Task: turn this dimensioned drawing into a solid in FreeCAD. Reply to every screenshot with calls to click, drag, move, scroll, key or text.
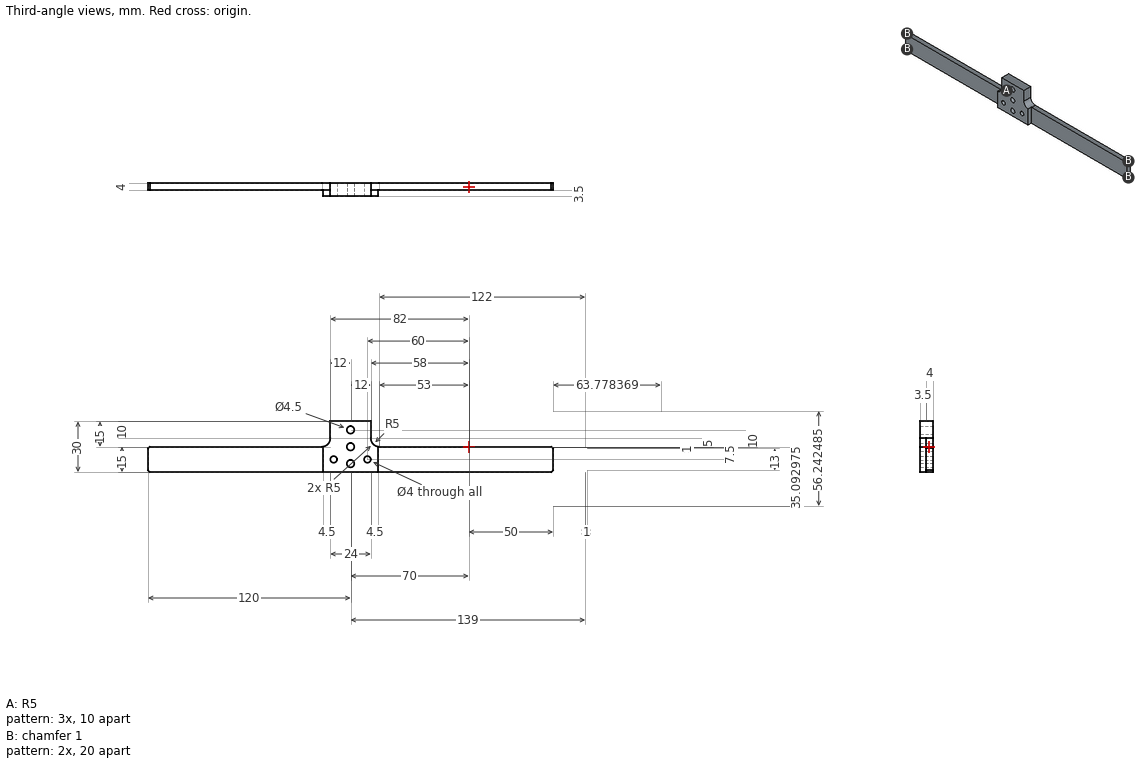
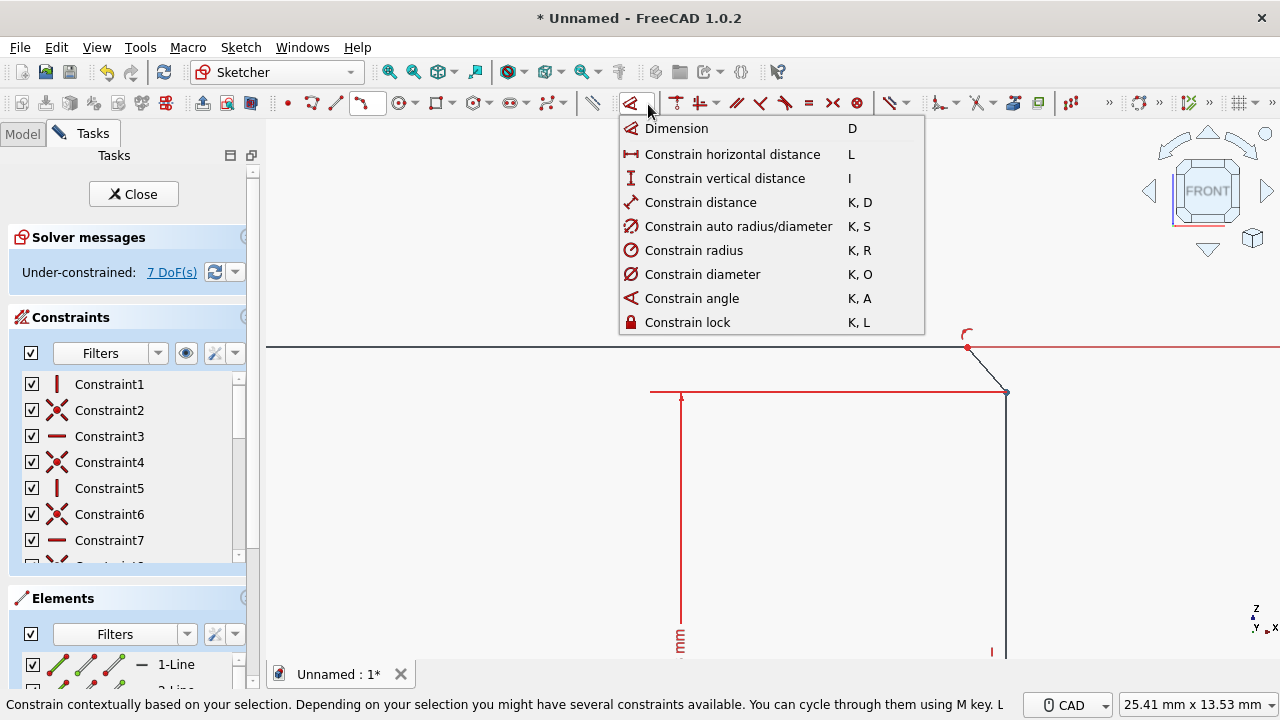
click(772, 178)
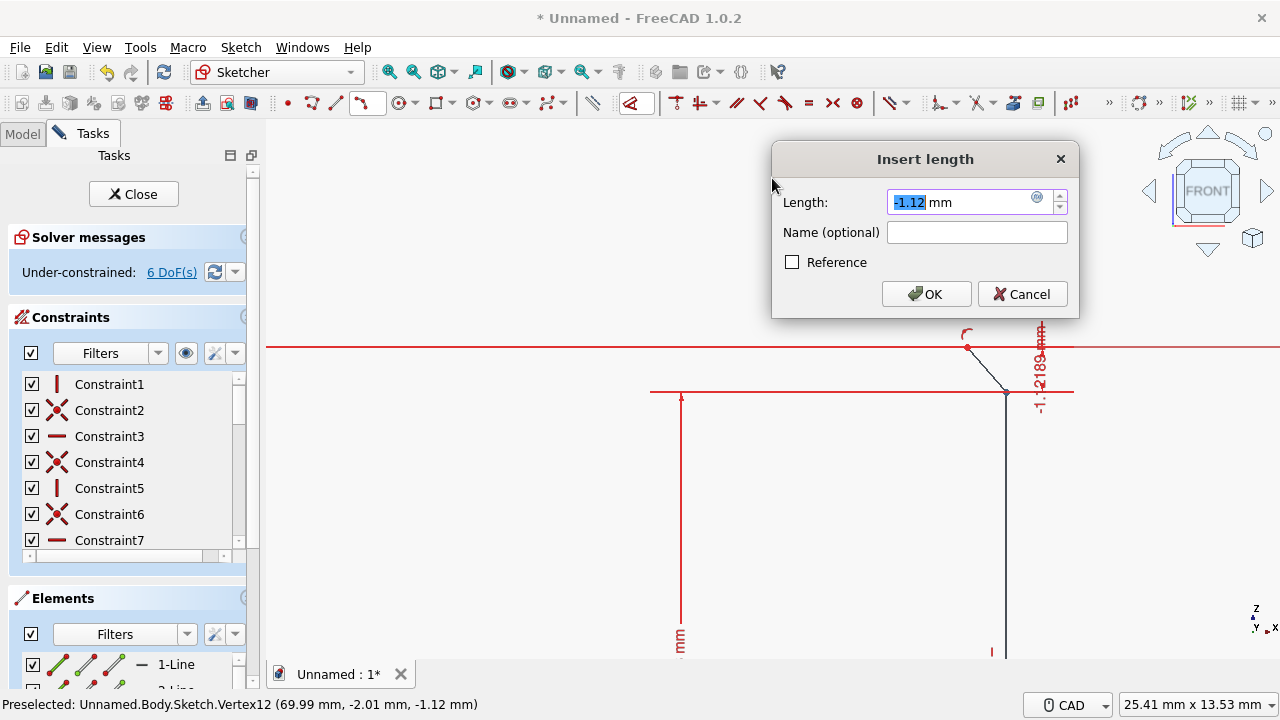
text(-1)
key(Return)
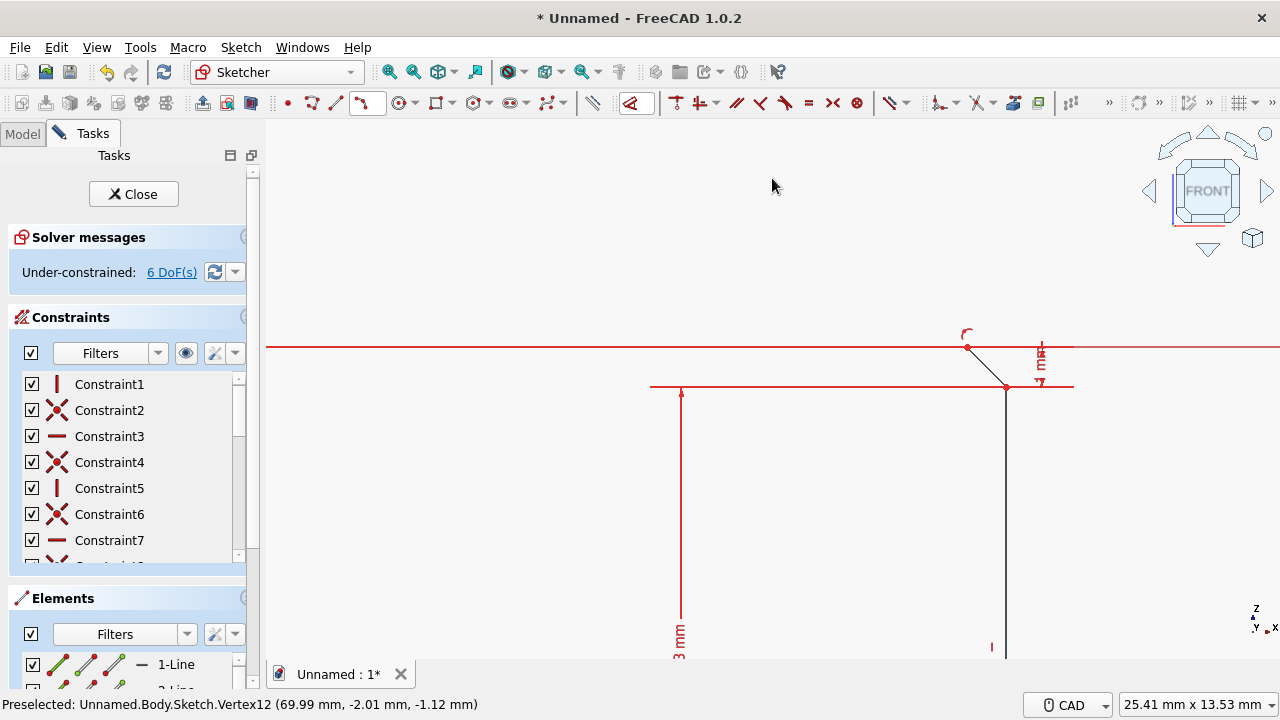
scroll(1015, 394, down, 11)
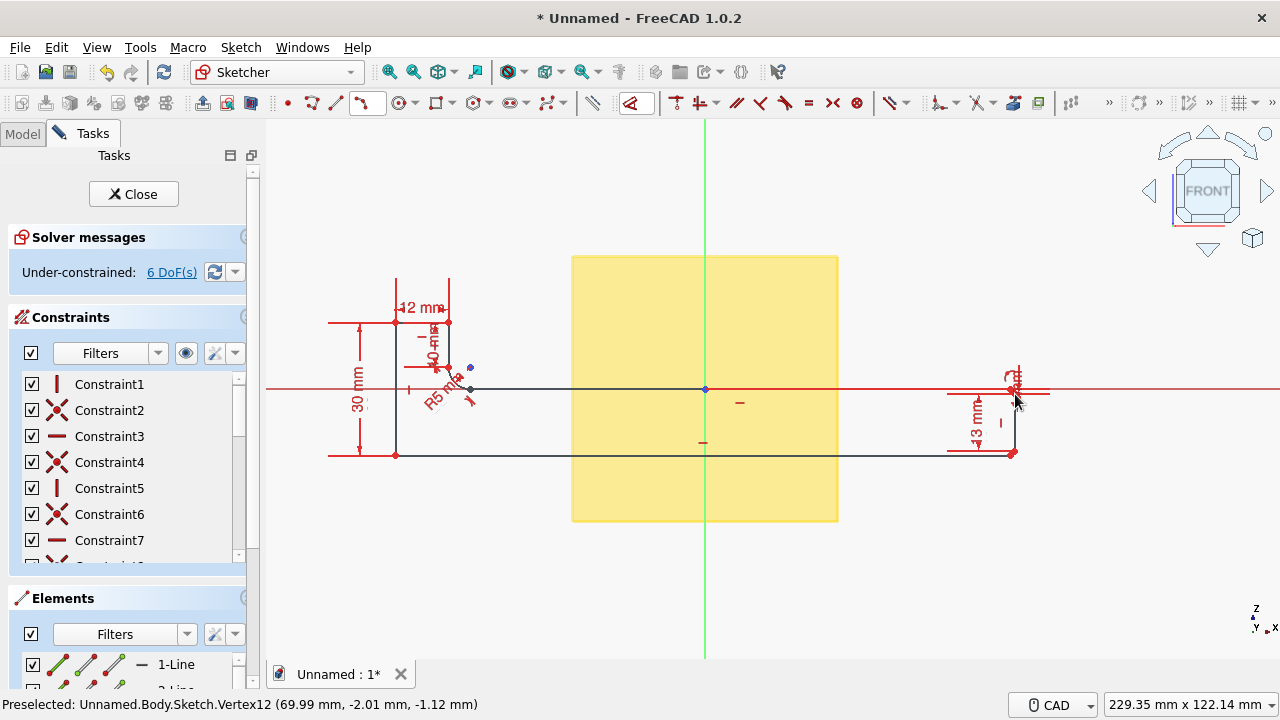
scroll(1012, 454, up, 11)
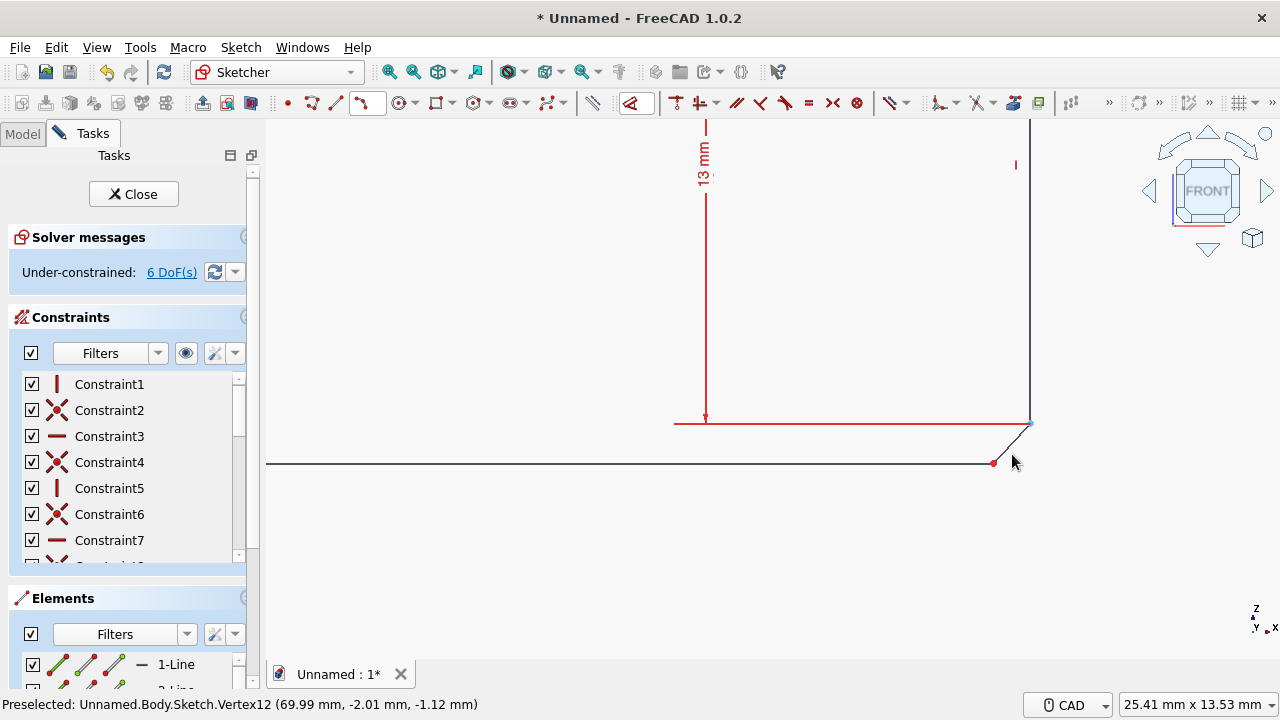
click(1005, 452)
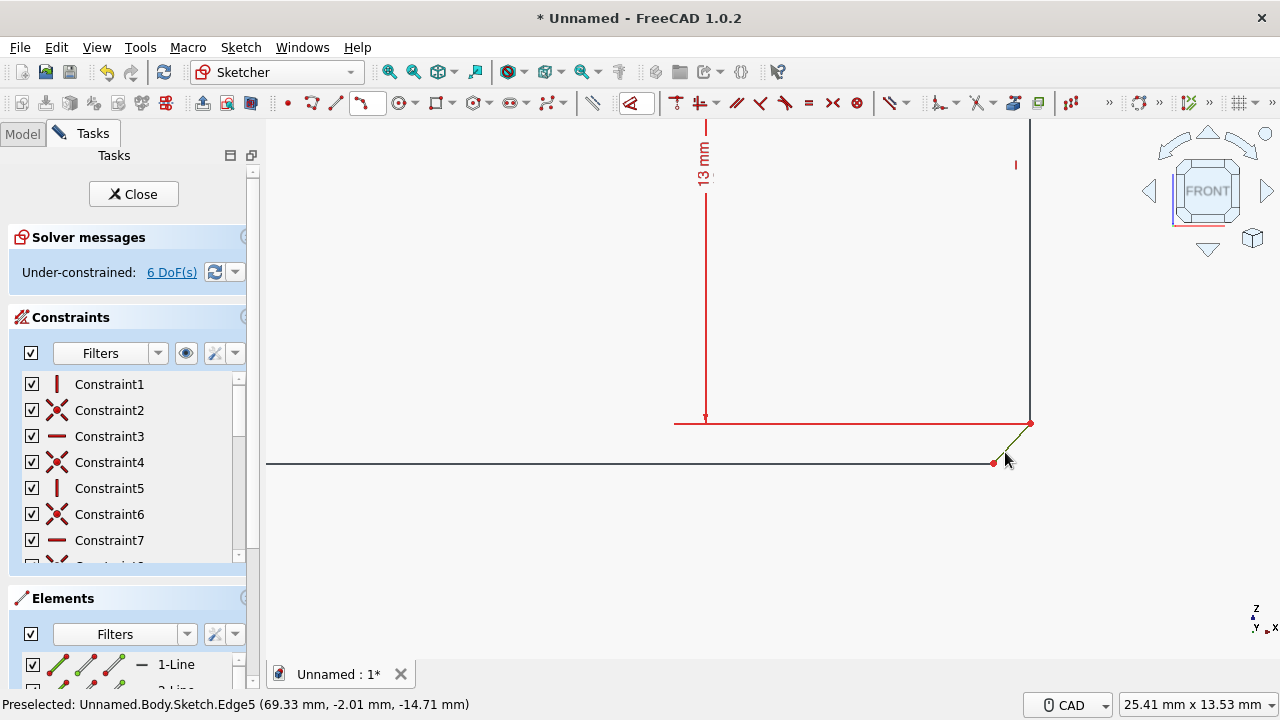
key(l)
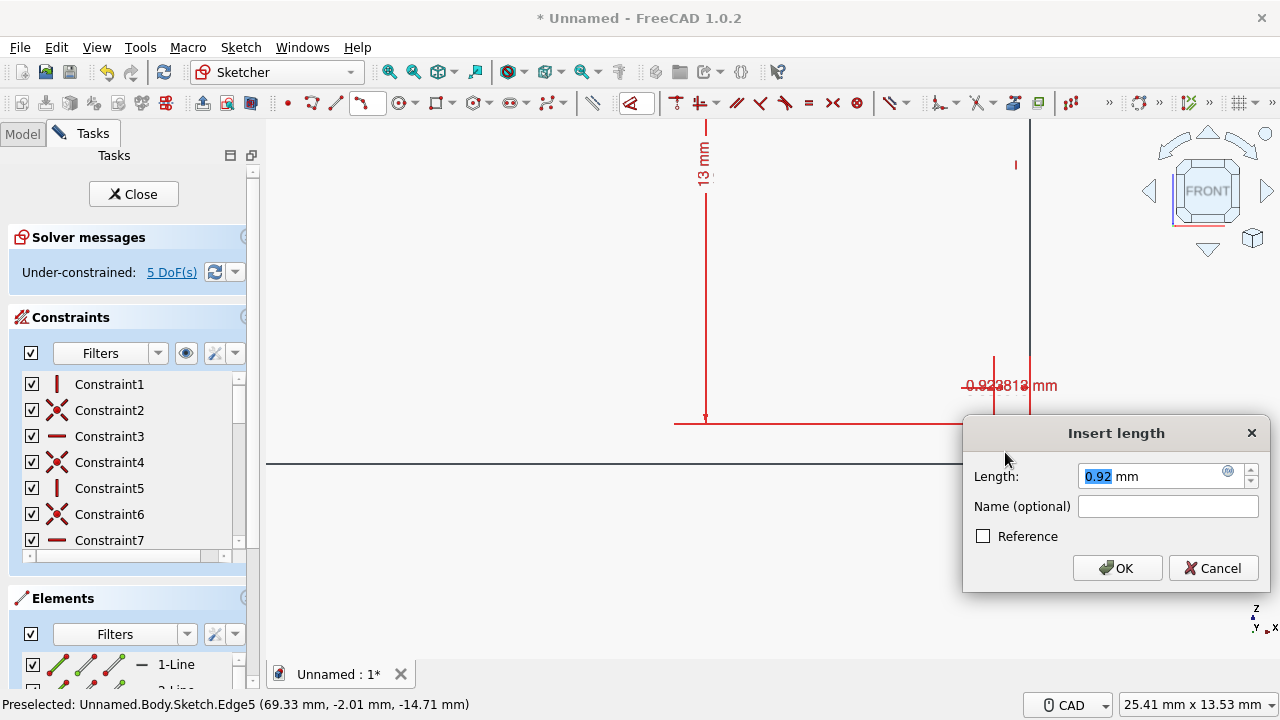
text(1)
key(Return)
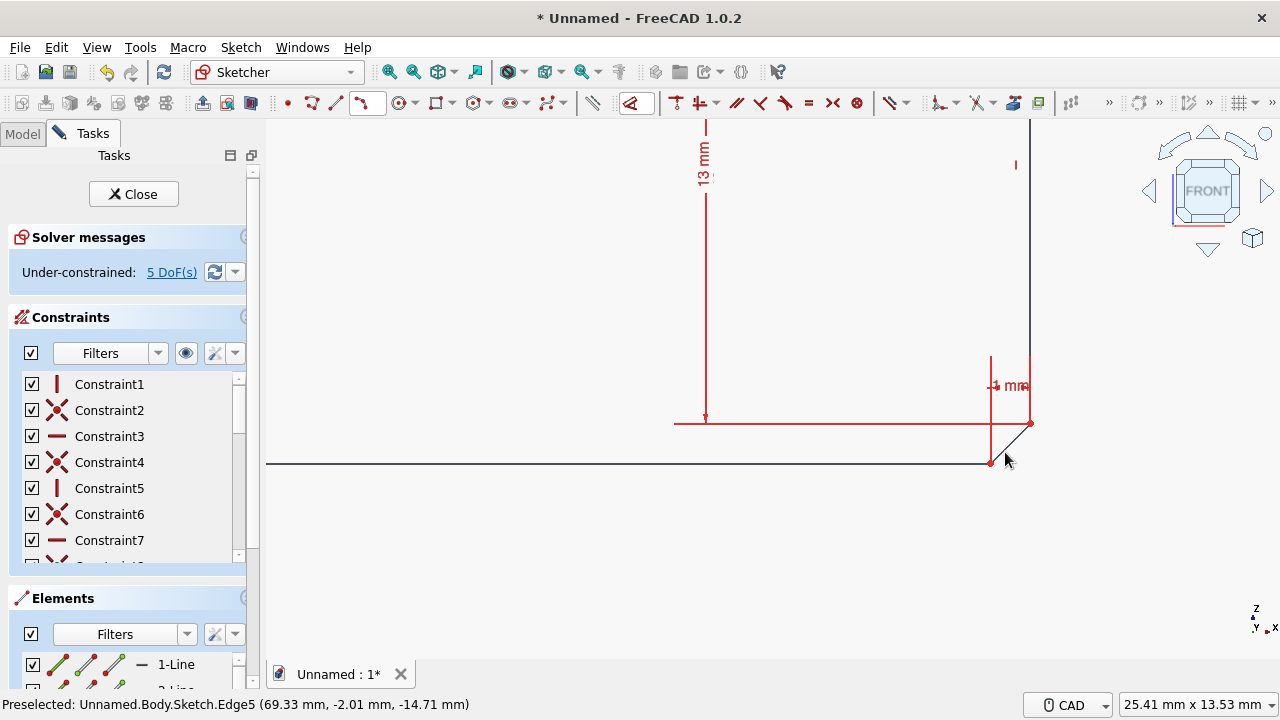
scroll(1012, 454, down, 11)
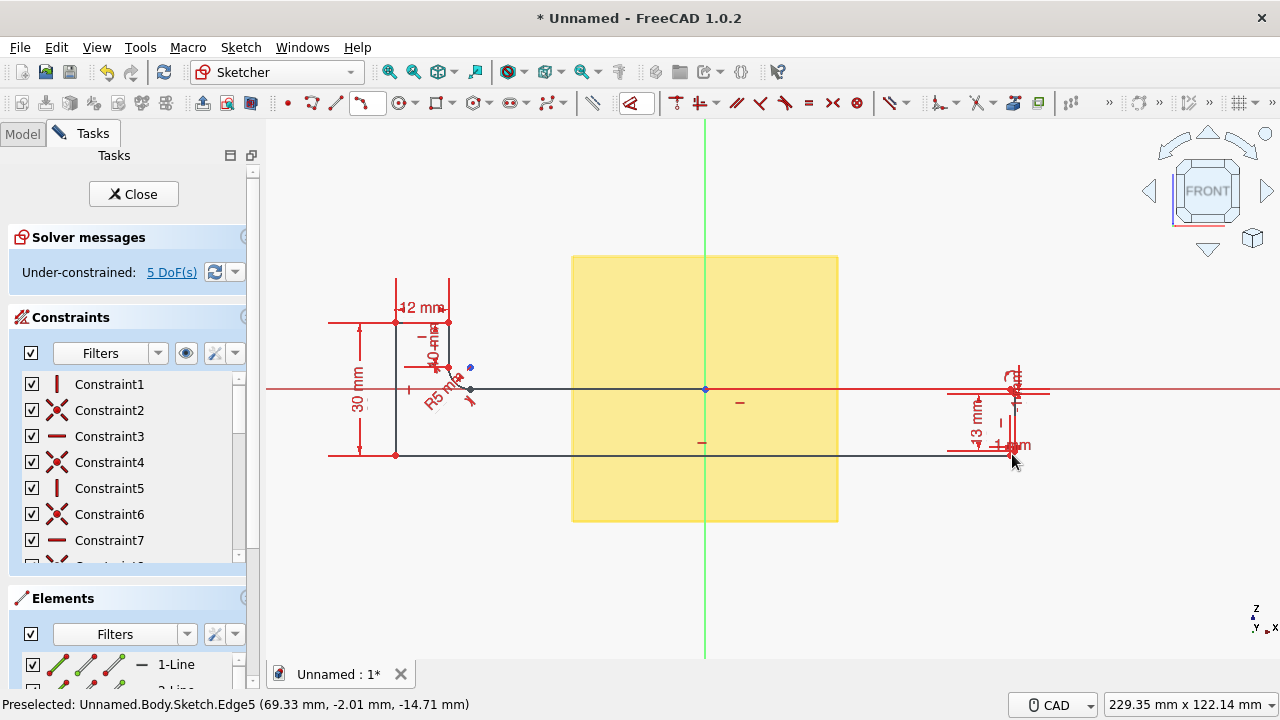
scroll(1013, 392, up, 11)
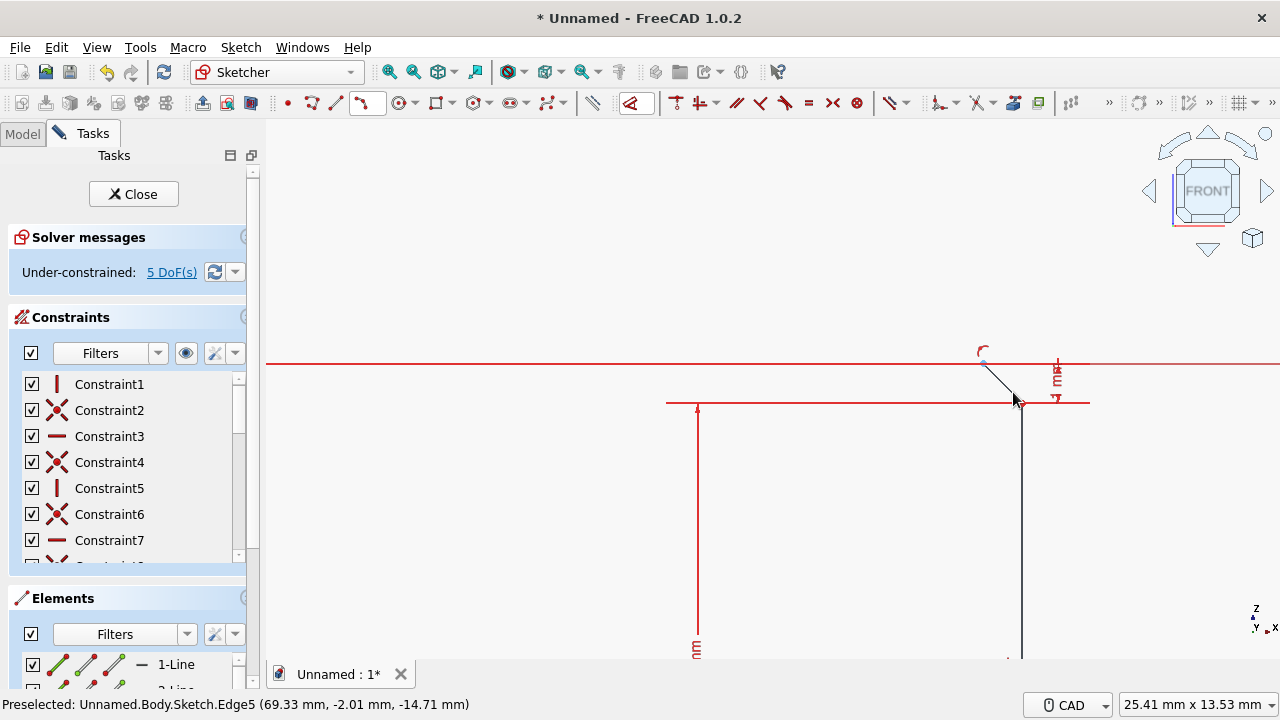
click(1011, 391)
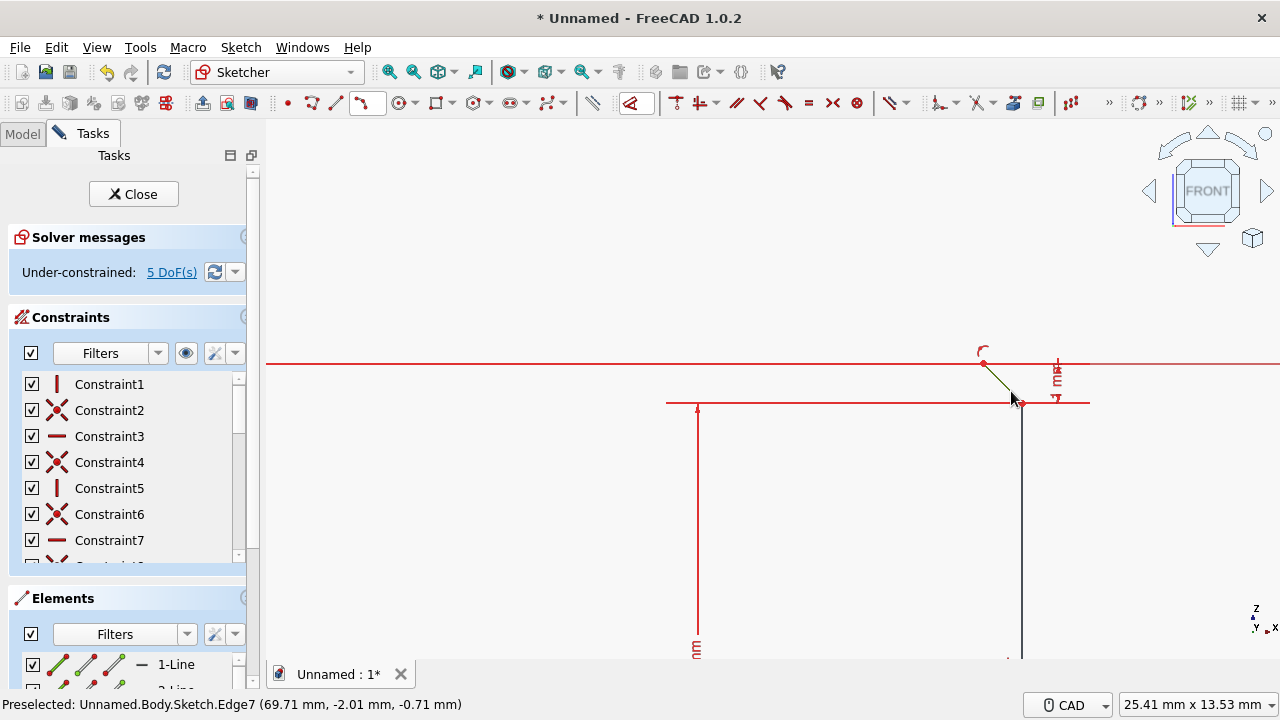
key(l)